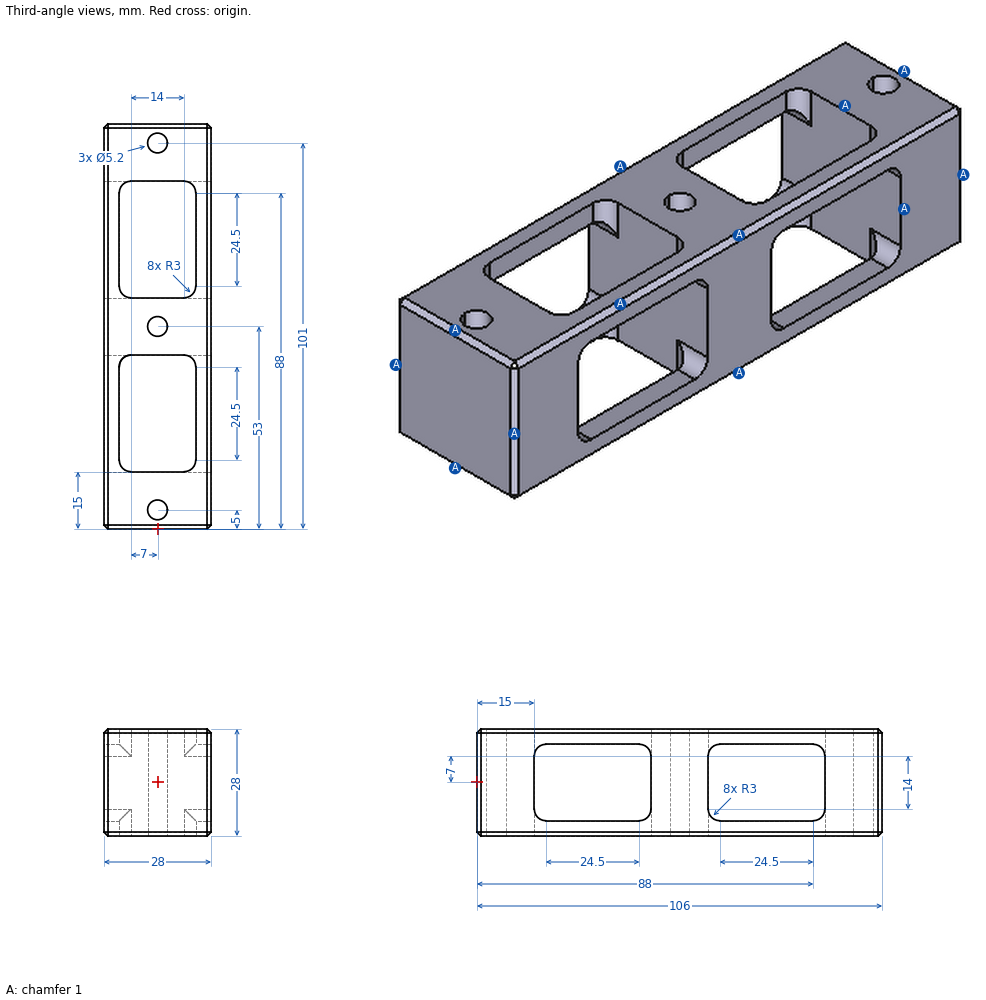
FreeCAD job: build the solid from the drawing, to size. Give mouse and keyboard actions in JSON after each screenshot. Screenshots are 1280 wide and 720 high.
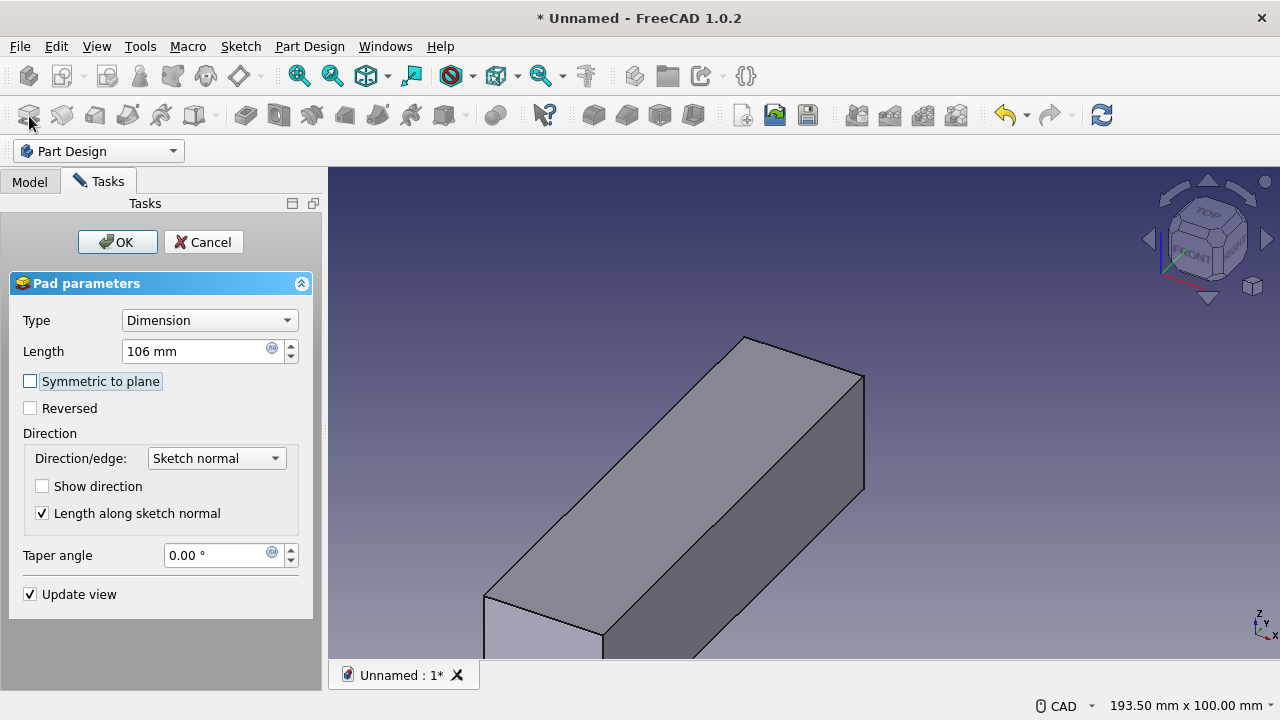
{"action": "left_click", "coordinate": [31, 408]}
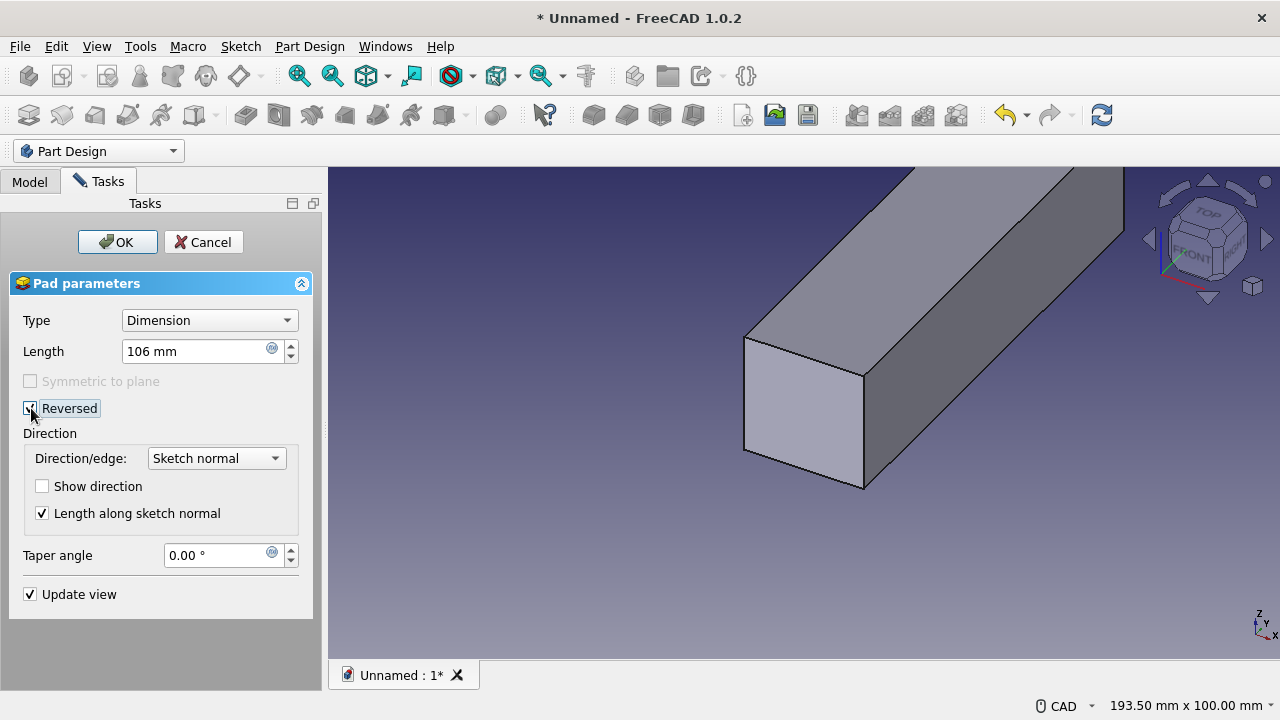
{"action": "left_click", "coordinate": [118, 242]}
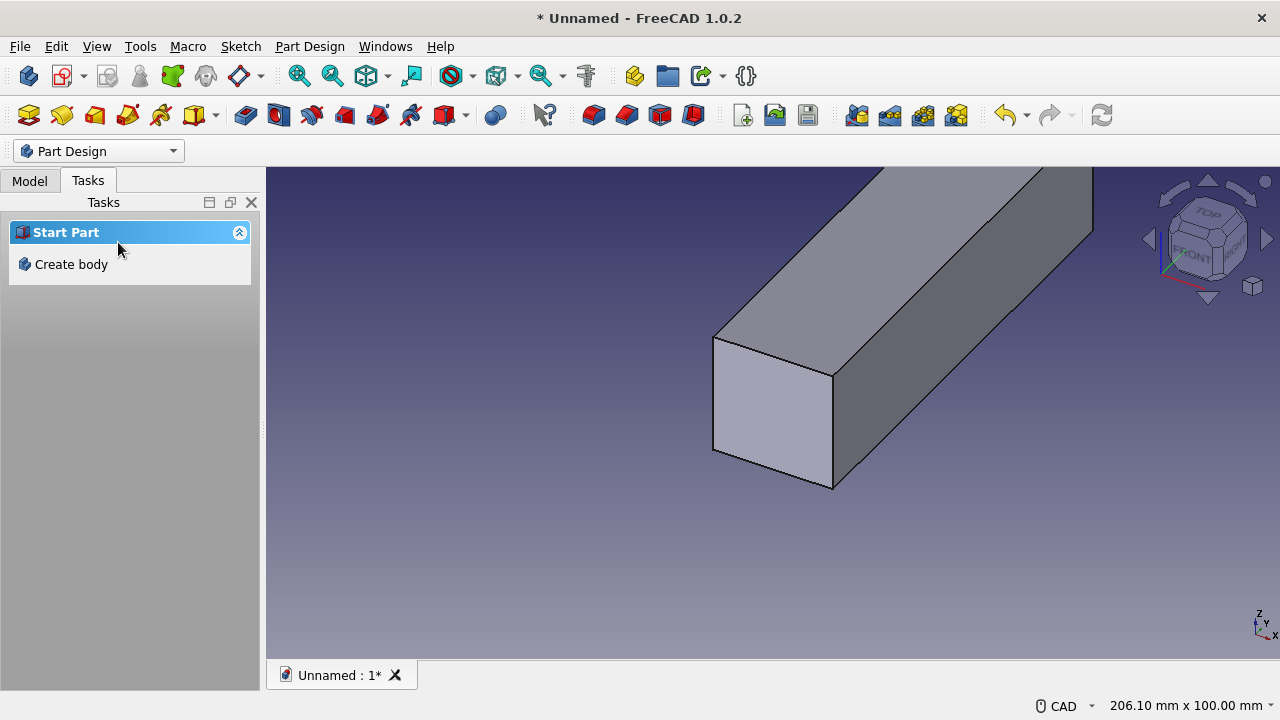
{"action": "left_click", "coordinate": [300, 76]}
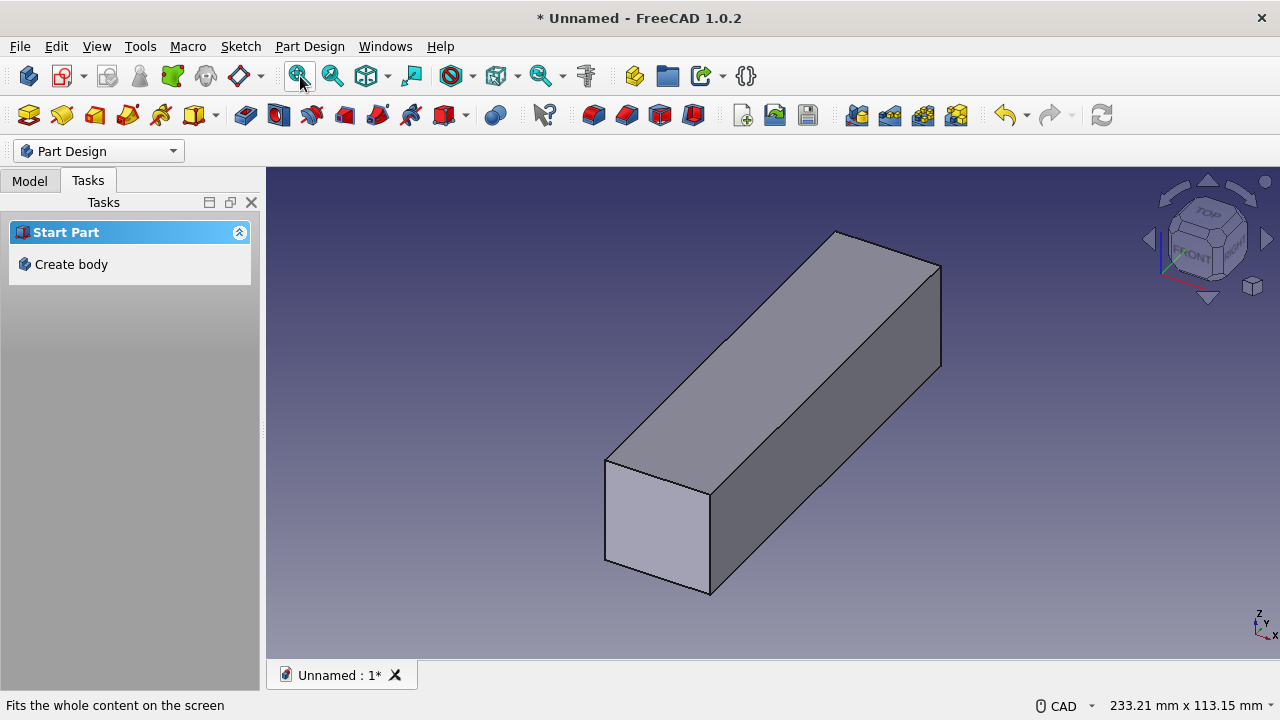
{"action": "left_click", "coordinate": [839, 297]}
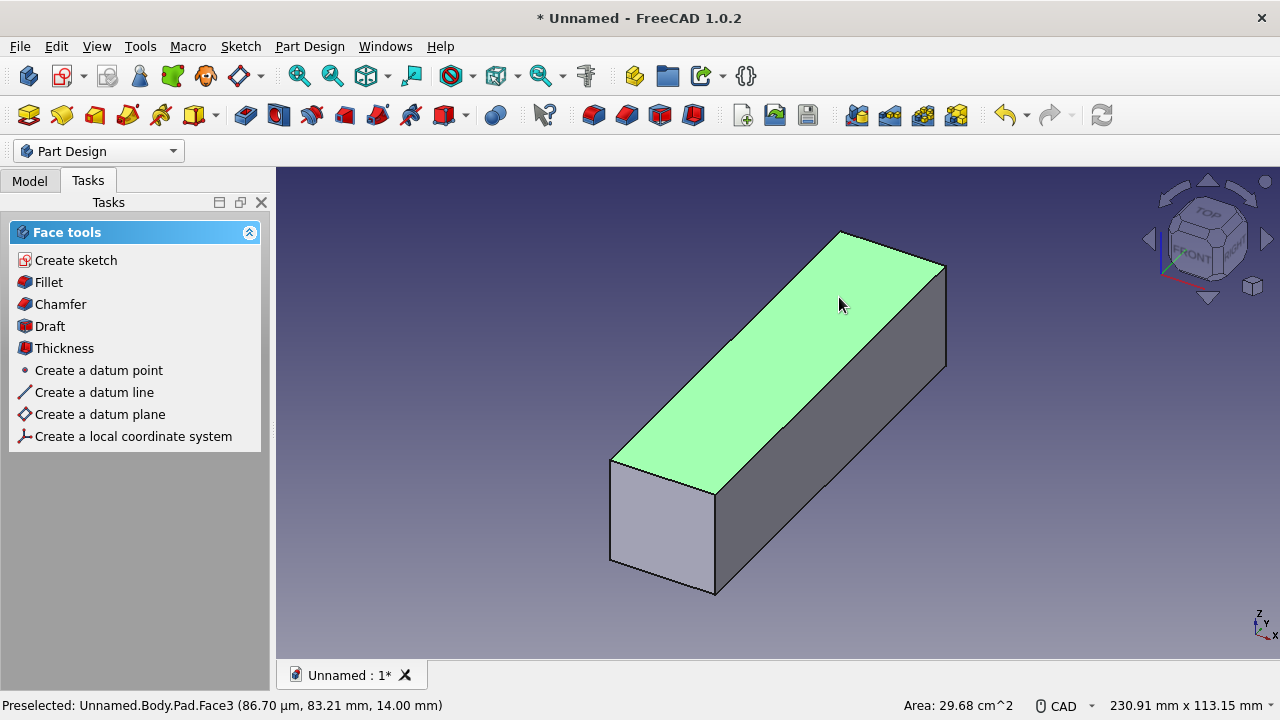
{"action": "left_click", "coordinate": [62, 76]}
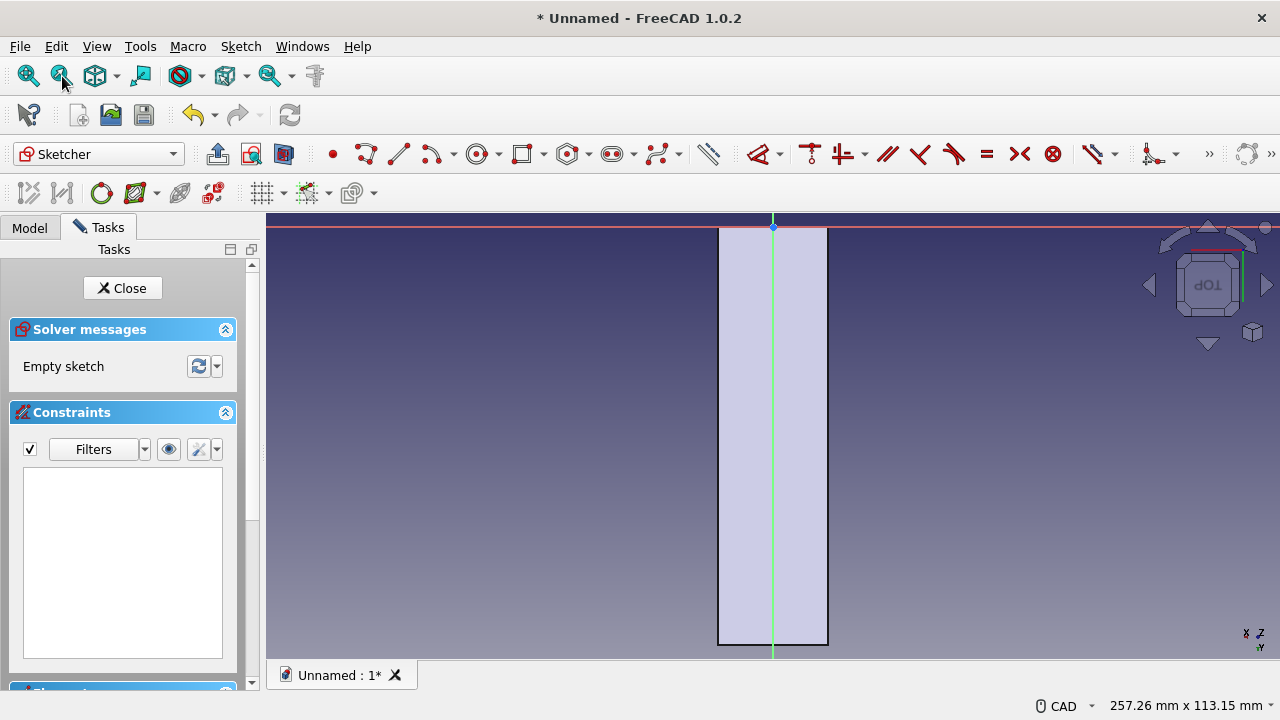
{"action": "scroll", "coordinate": [565, 446], "scroll_direction": "down", "scroll_amount": 2}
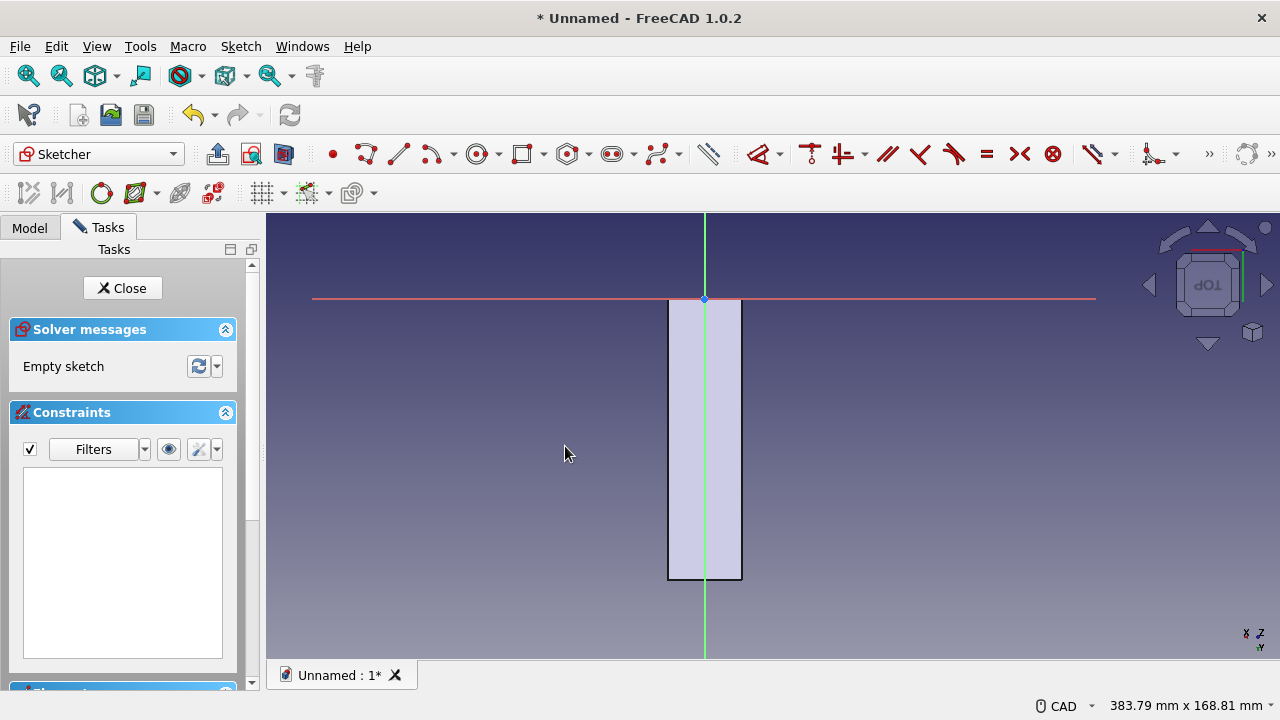
{"action": "left_click", "coordinate": [399, 154]}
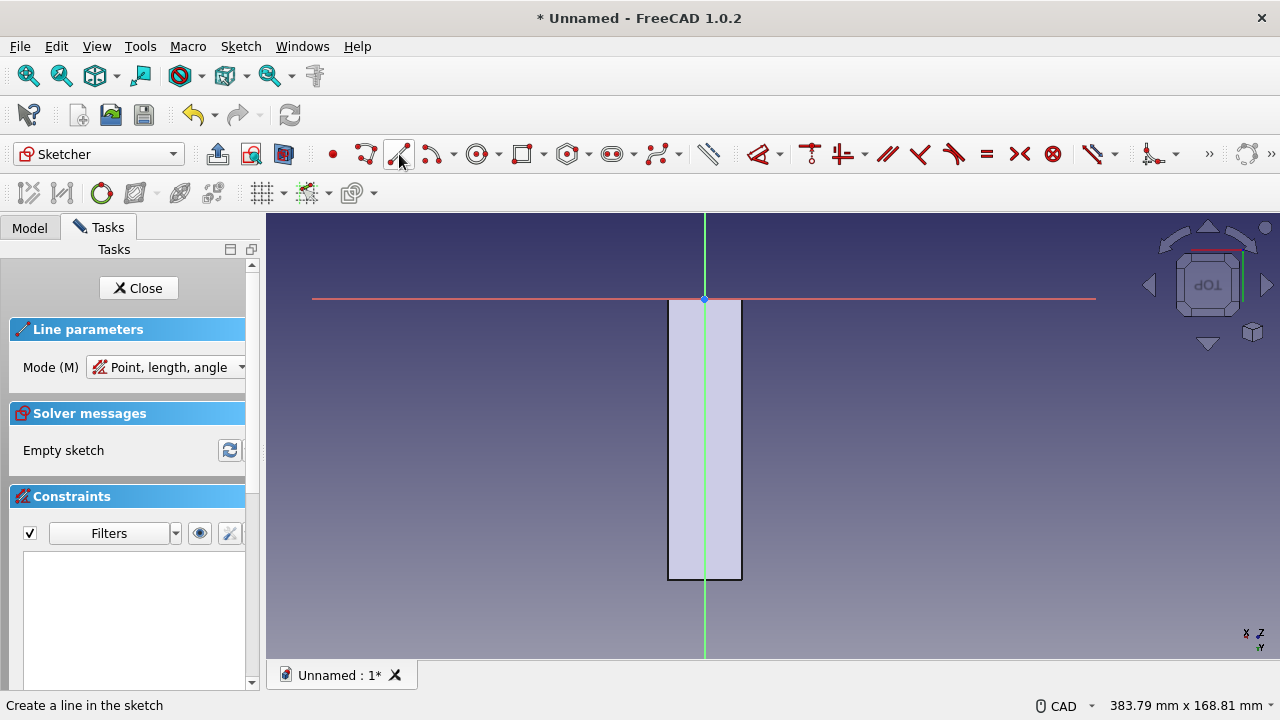
{"action": "left_click", "coordinate": [723, 459]}
{"action": "left_click", "coordinate": [686, 459]}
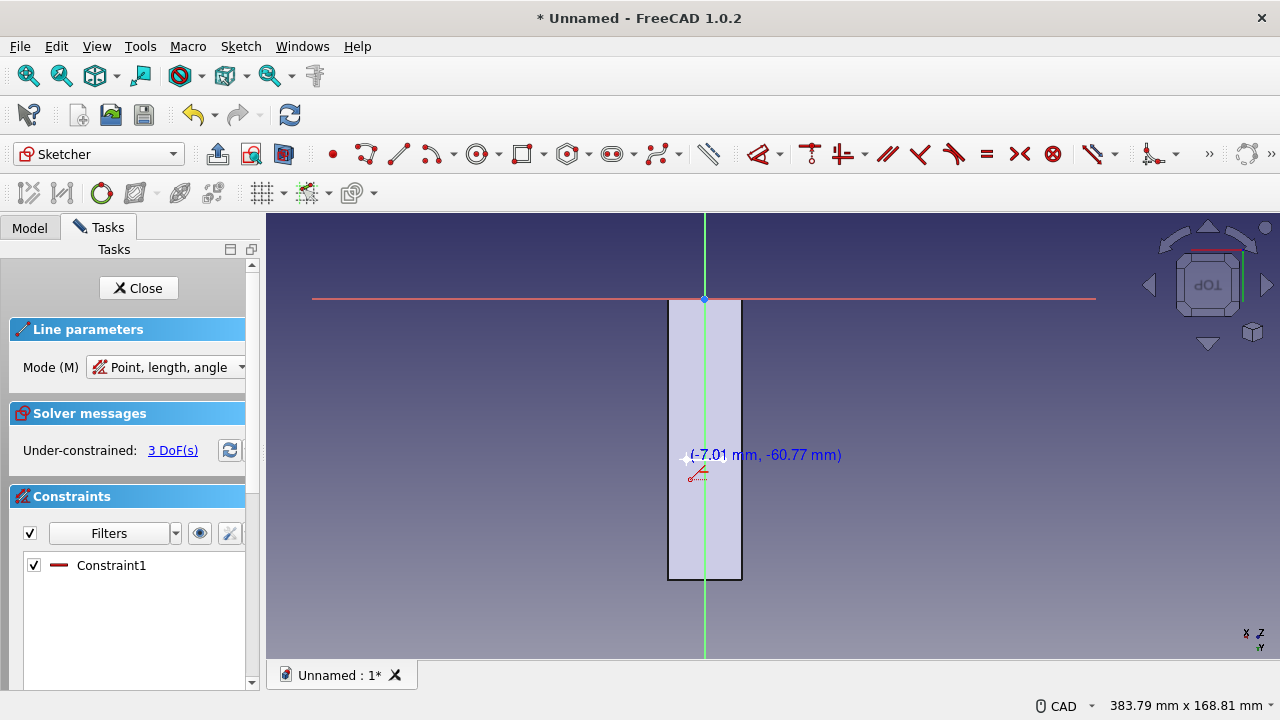
{"action": "scroll", "coordinate": [678, 467], "scroll_direction": "up", "scroll_amount": 2}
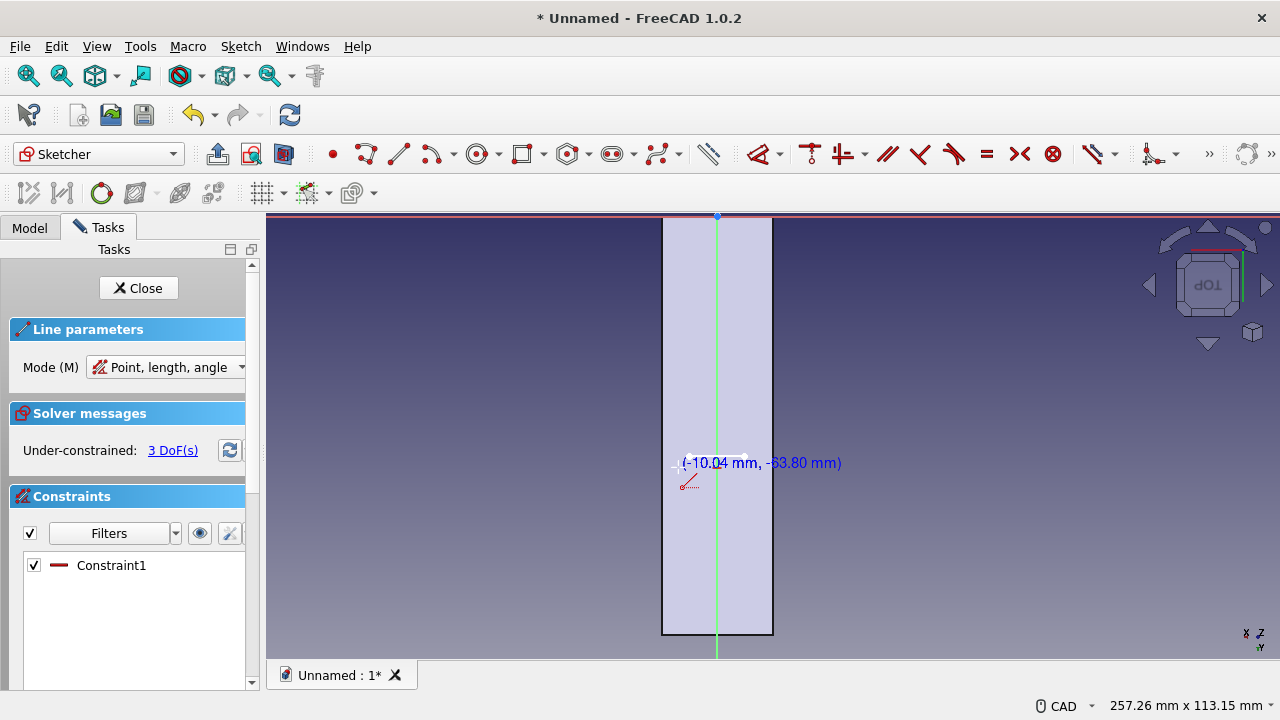
{"action": "left_click", "coordinate": [678, 467]}
{"action": "left_click", "coordinate": [678, 564]}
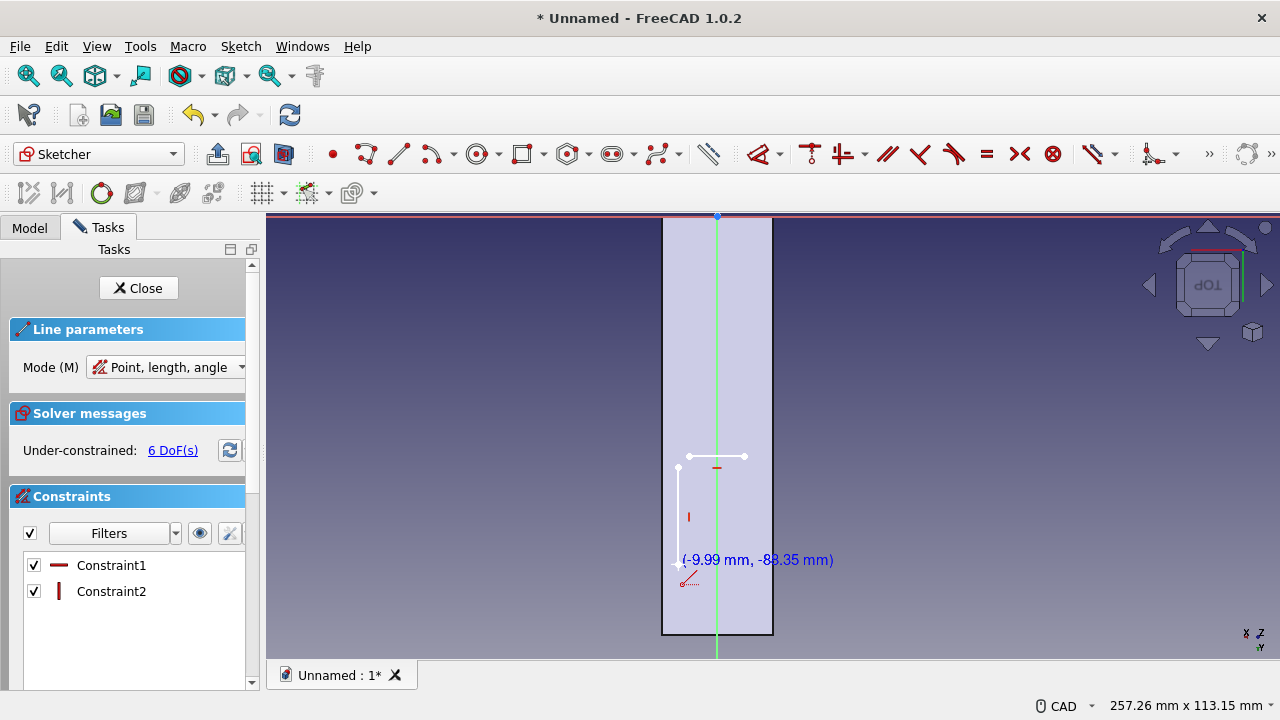
{"action": "left_click", "coordinate": [690, 575]}
{"action": "left_click", "coordinate": [745, 575]}